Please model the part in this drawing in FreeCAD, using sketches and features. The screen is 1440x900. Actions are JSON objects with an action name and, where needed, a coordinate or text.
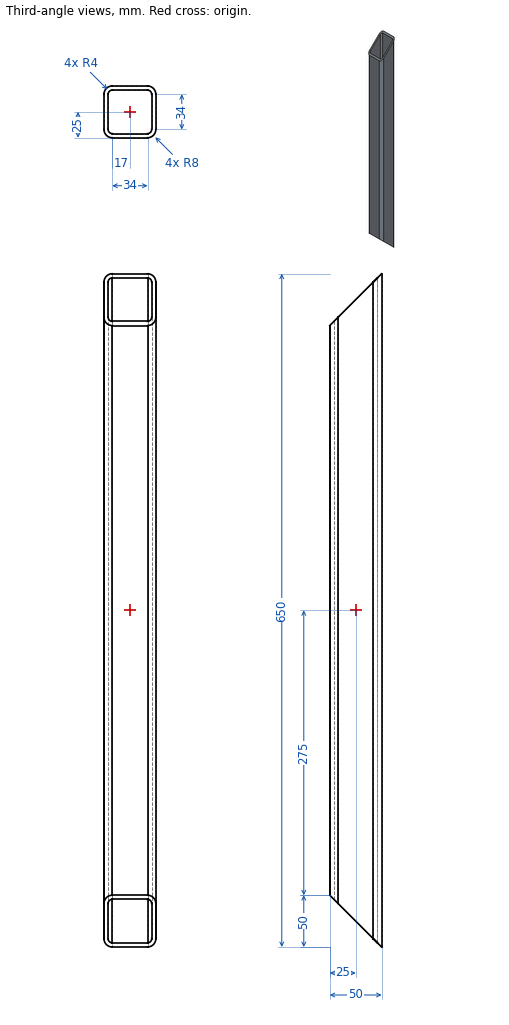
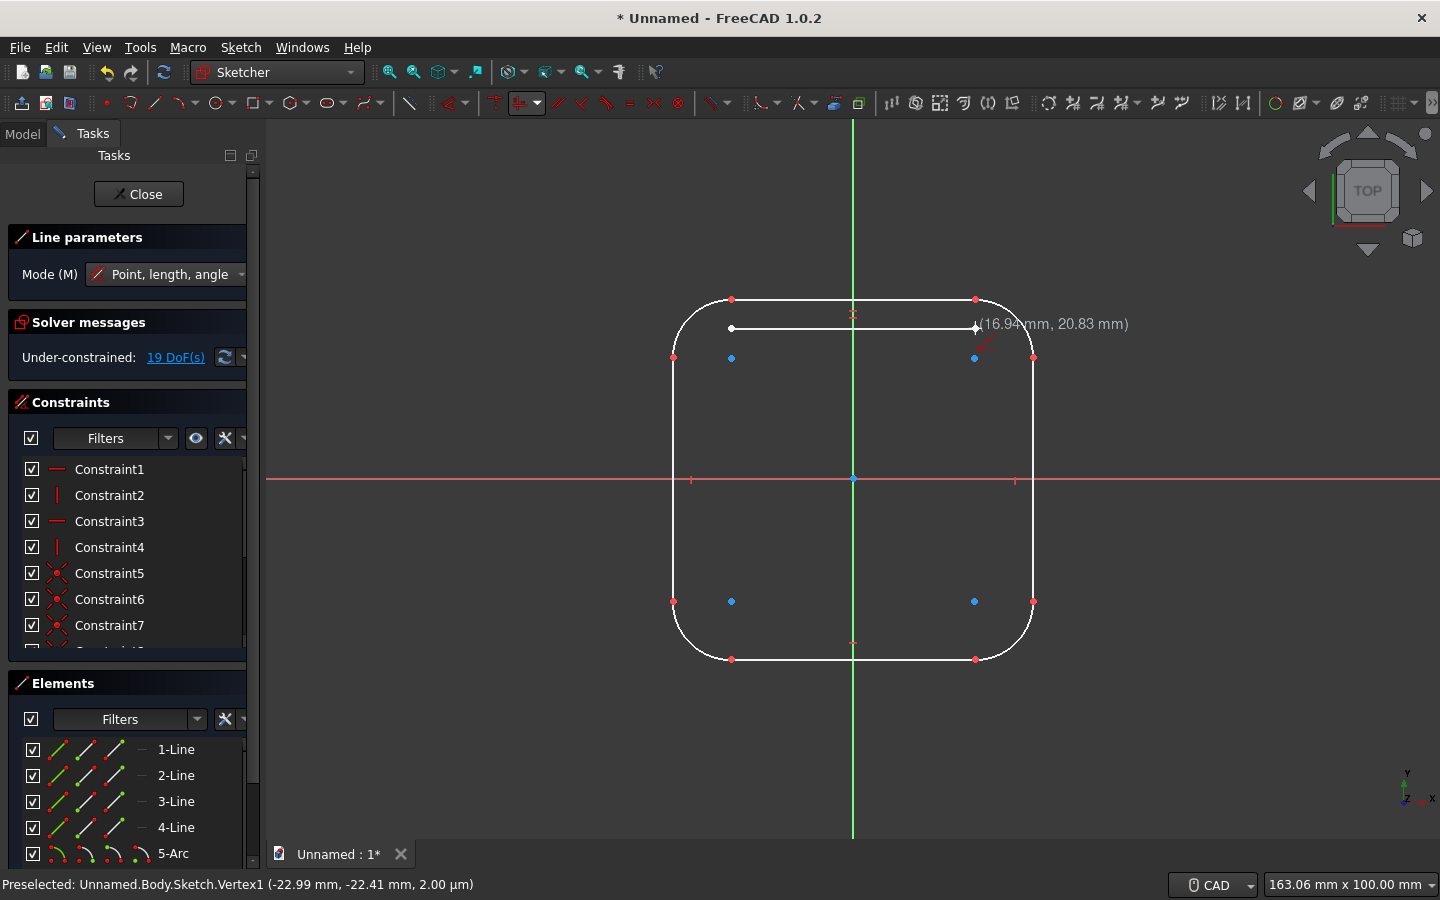
{"action": "left_click", "coordinate": [1004, 357]}
{"action": "left_click", "coordinate": [1004, 601]}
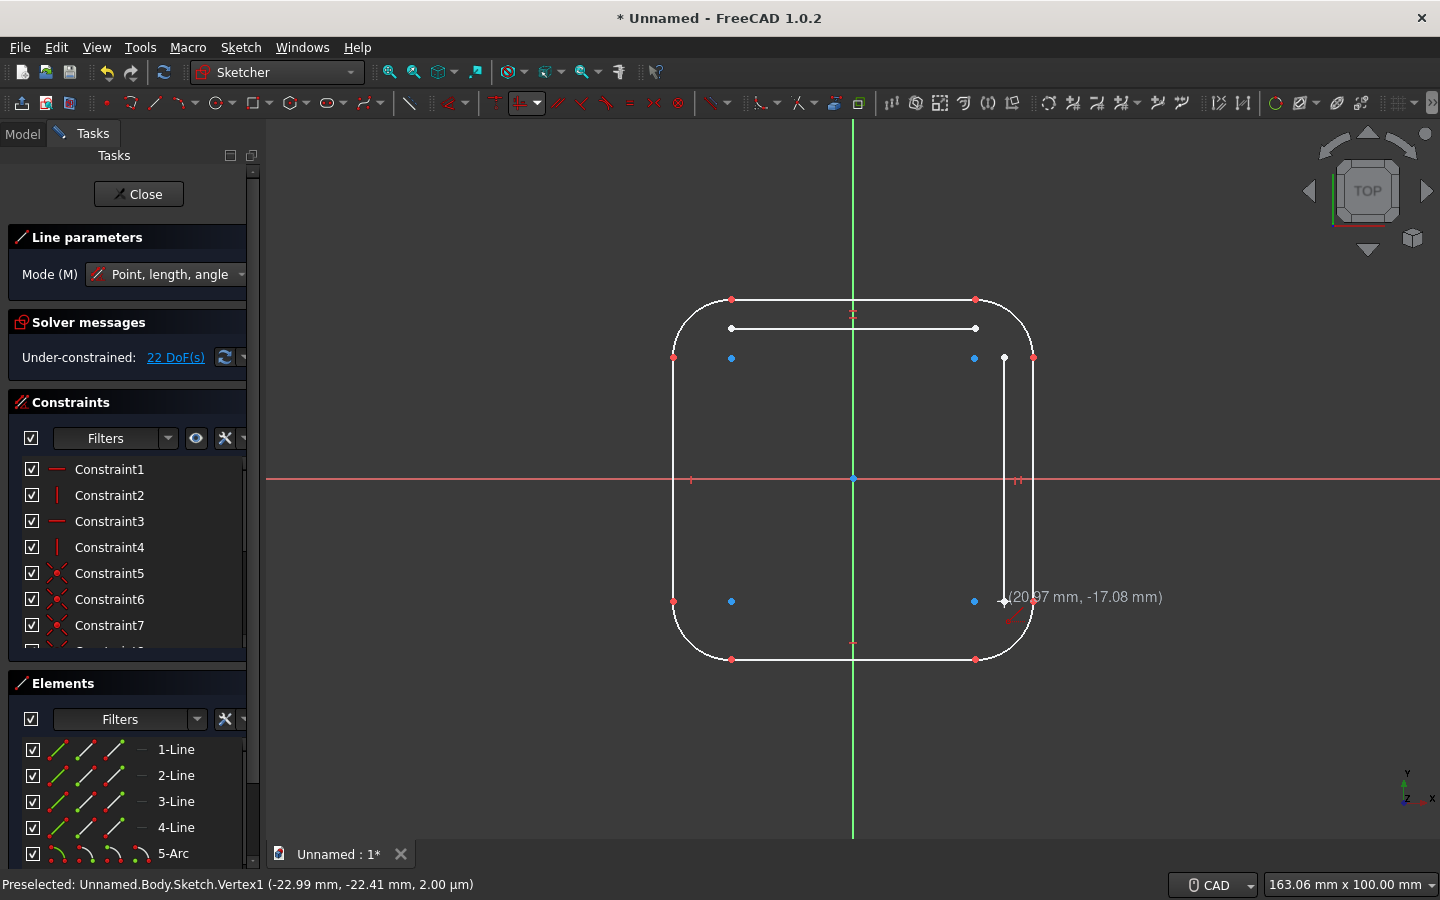
{"action": "left_click", "coordinate": [975, 630]}
{"action": "left_click", "coordinate": [731, 630]}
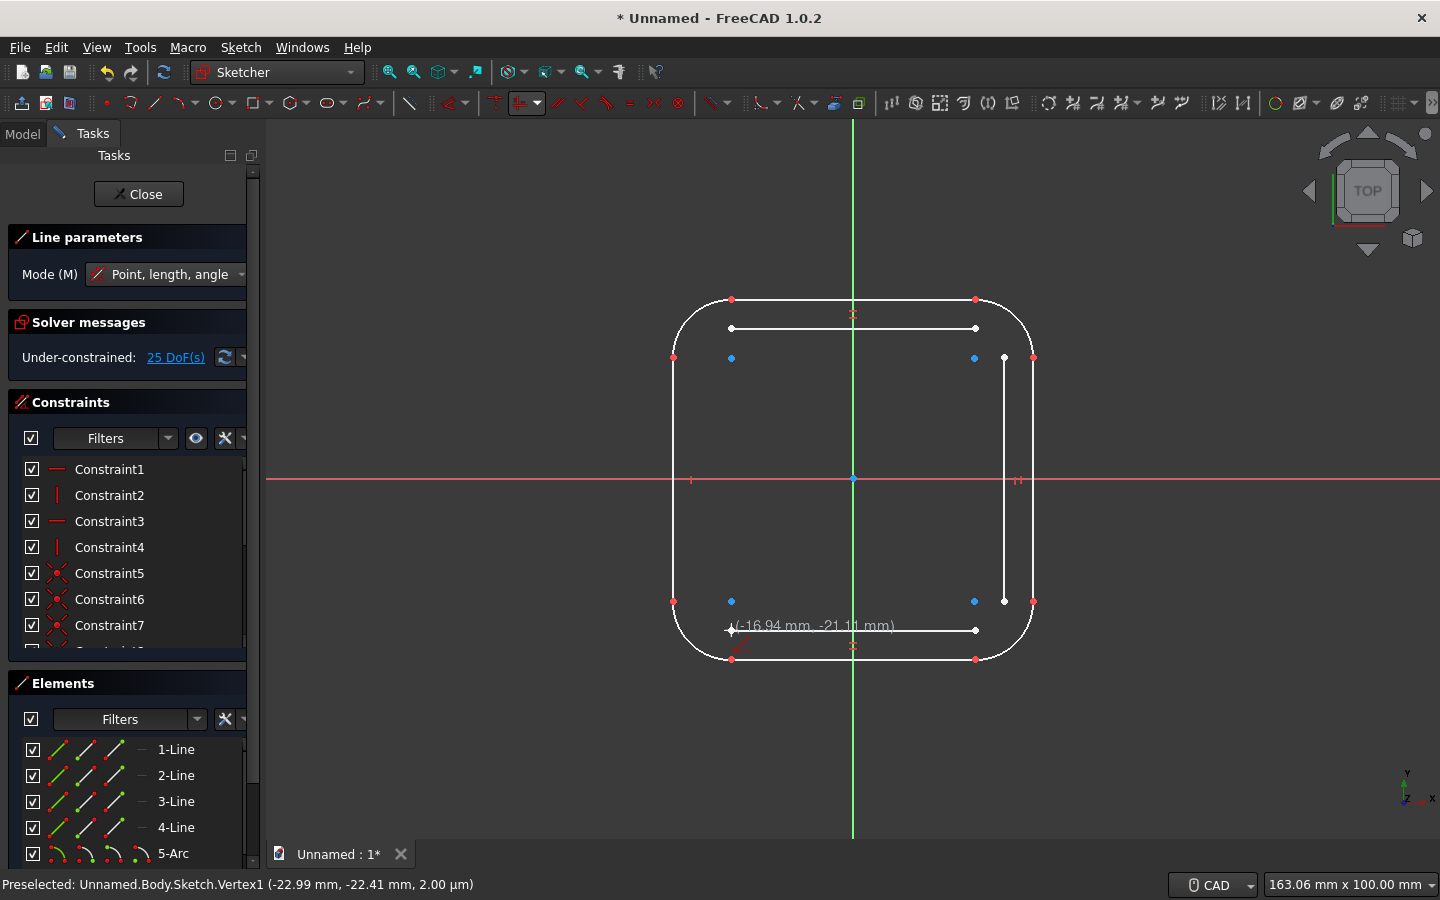
{"action": "left_click", "coordinate": [702, 601]}
{"action": "left_click", "coordinate": [702, 357]}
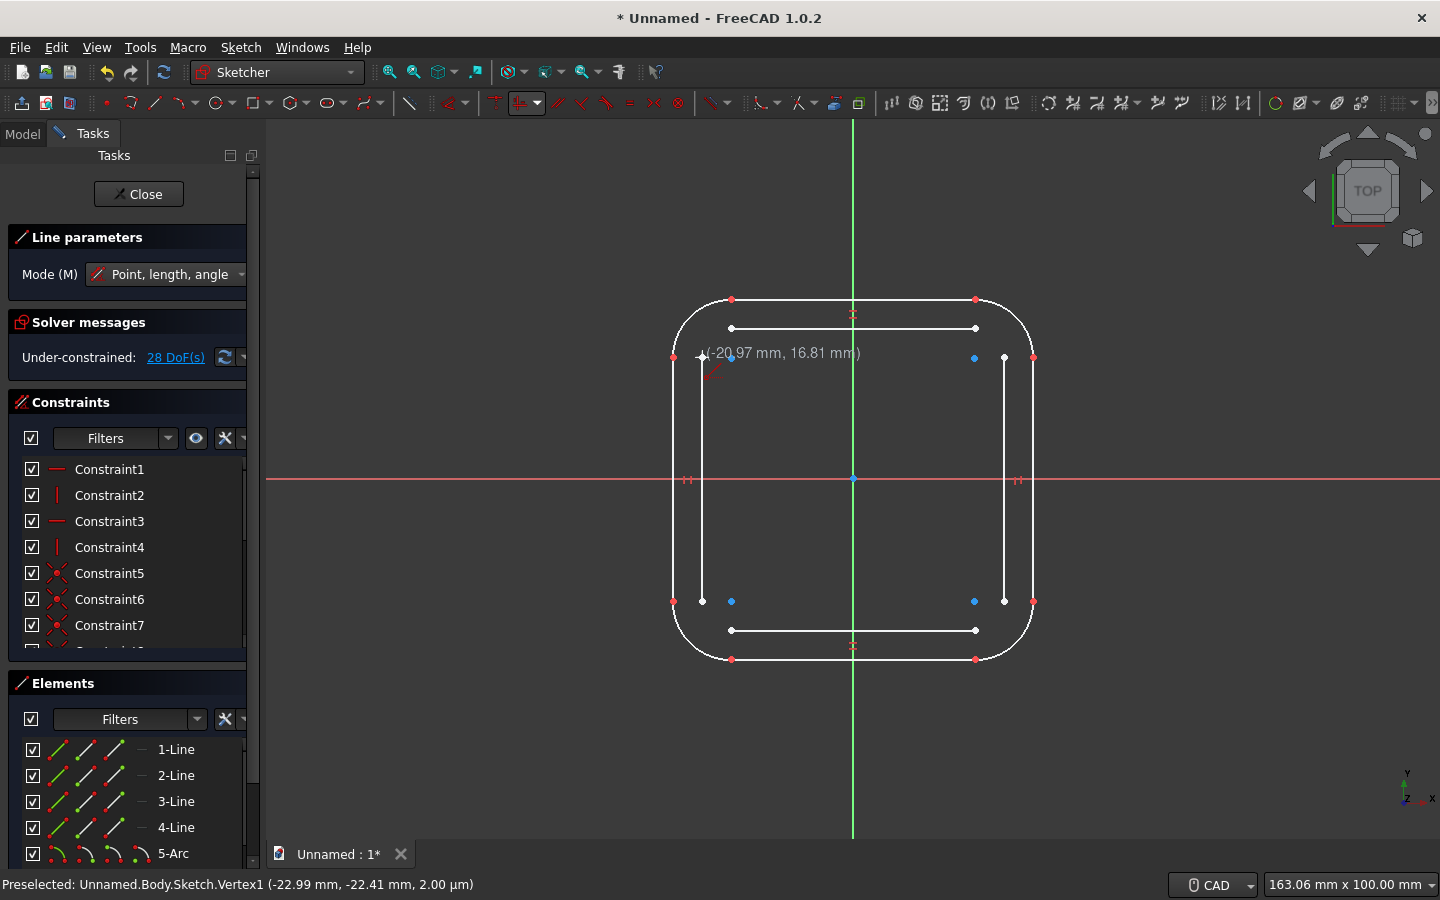
{"action": "key", "text": "g 3 a"}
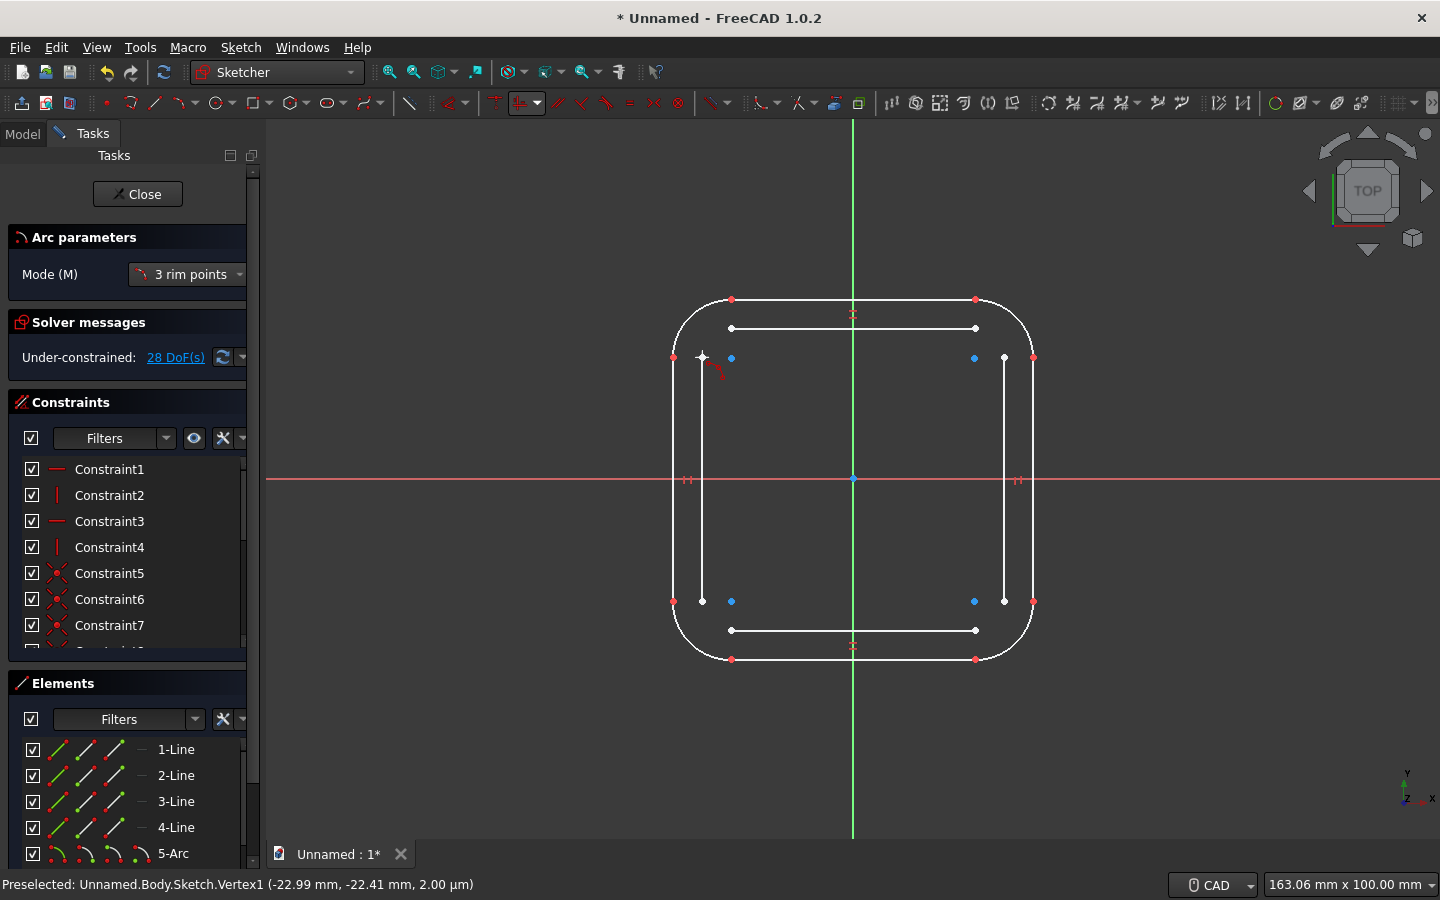
{"action": "left_click", "coordinate": [975, 329]}
{"action": "left_click", "coordinate": [1004, 358]}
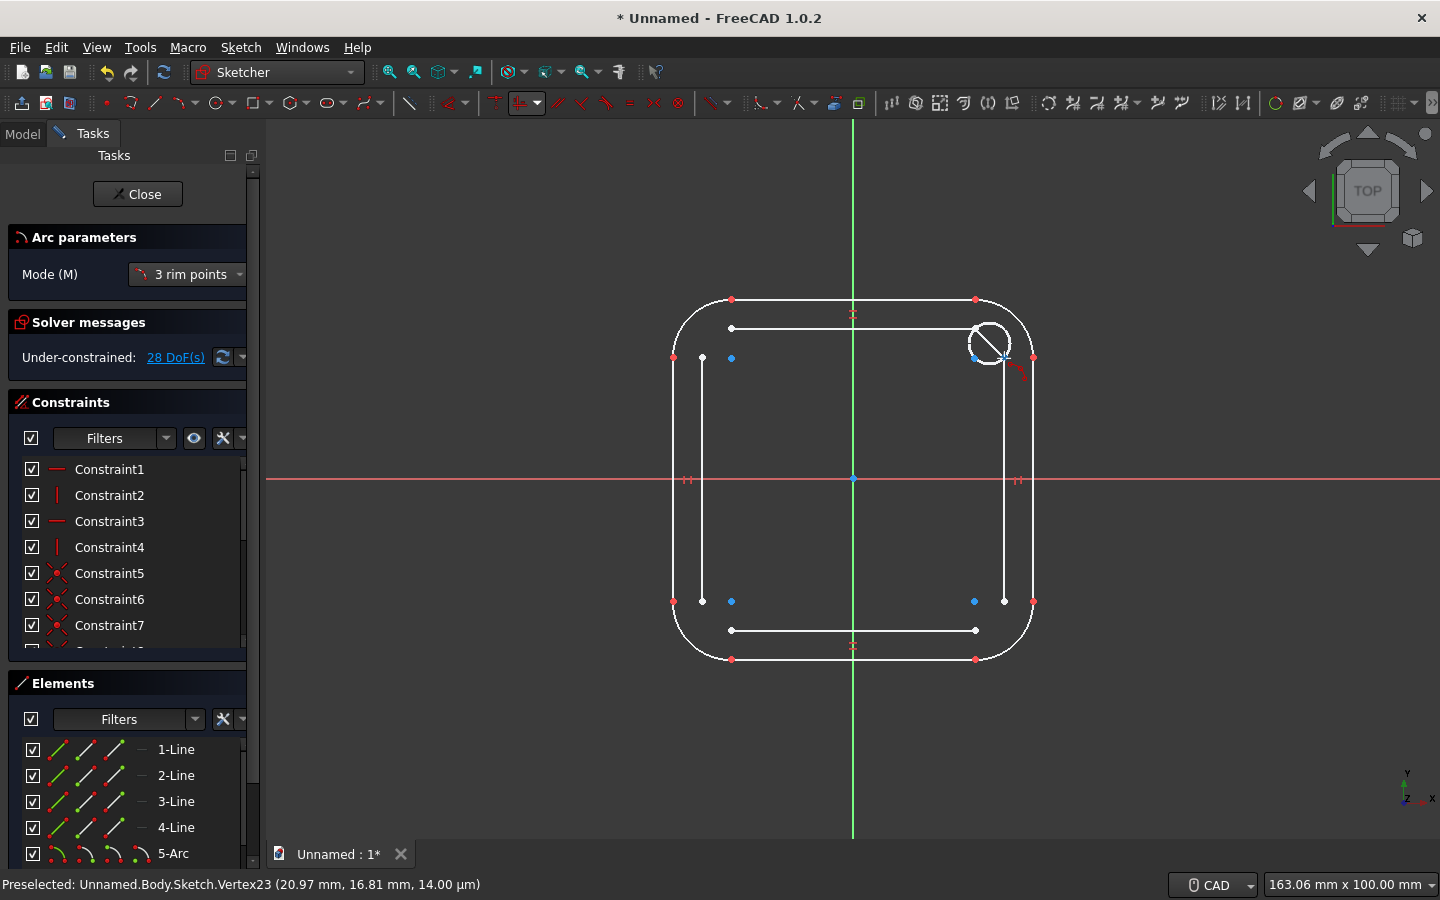
{"action": "scroll", "coordinate": [996, 336], "scroll_direction": "up", "scroll_amount": 4}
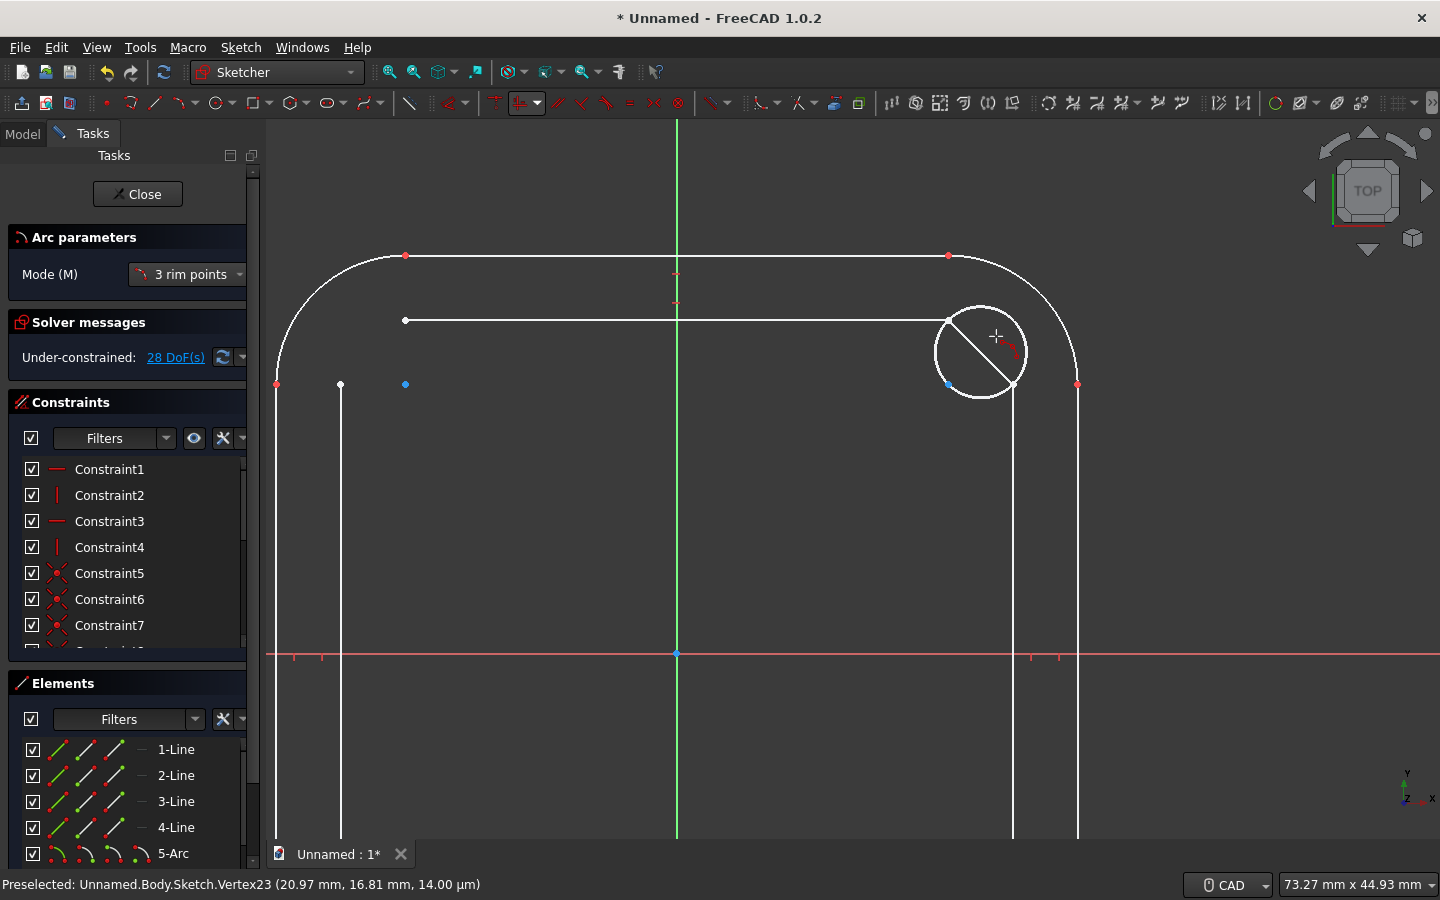
{"action": "left_click", "coordinate": [995, 336]}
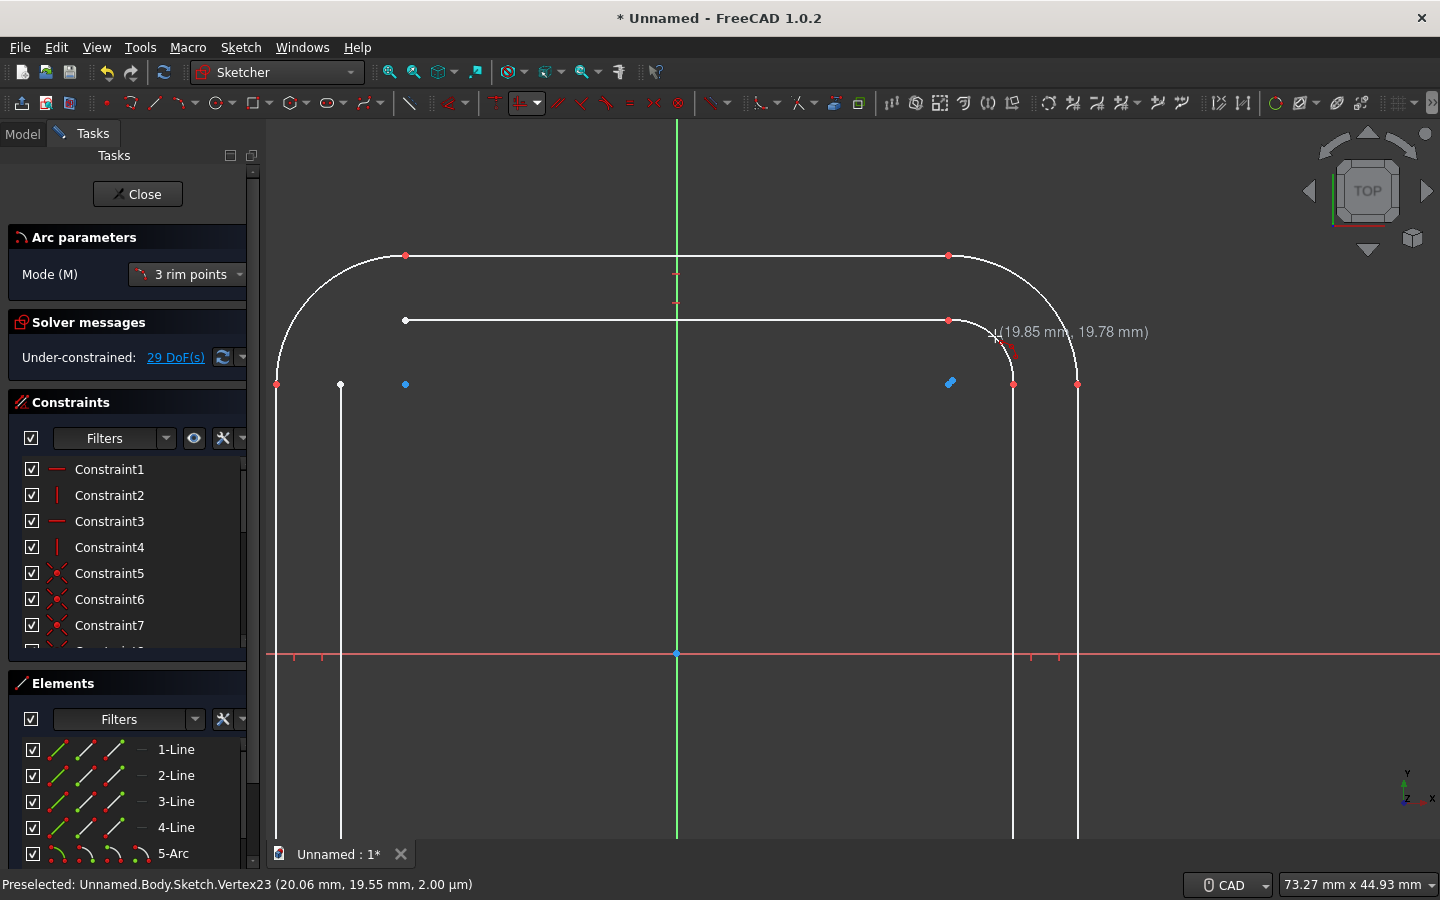
{"action": "scroll", "coordinate": [915, 266], "scroll_direction": "down", "scroll_amount": 3}